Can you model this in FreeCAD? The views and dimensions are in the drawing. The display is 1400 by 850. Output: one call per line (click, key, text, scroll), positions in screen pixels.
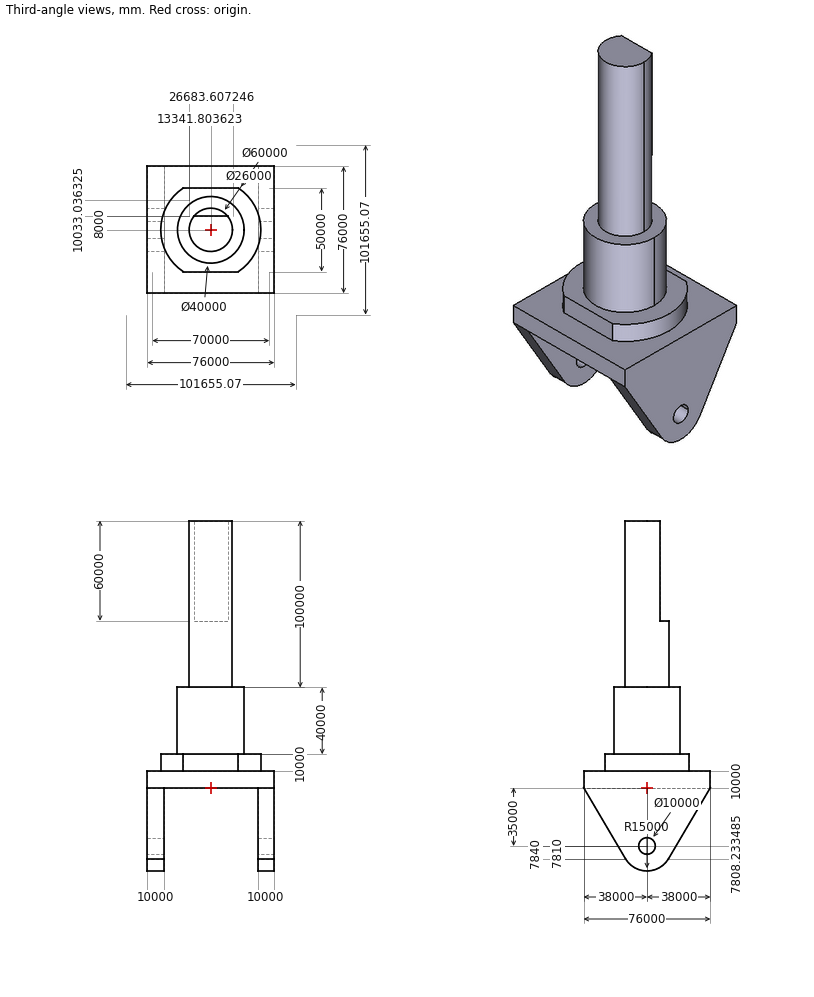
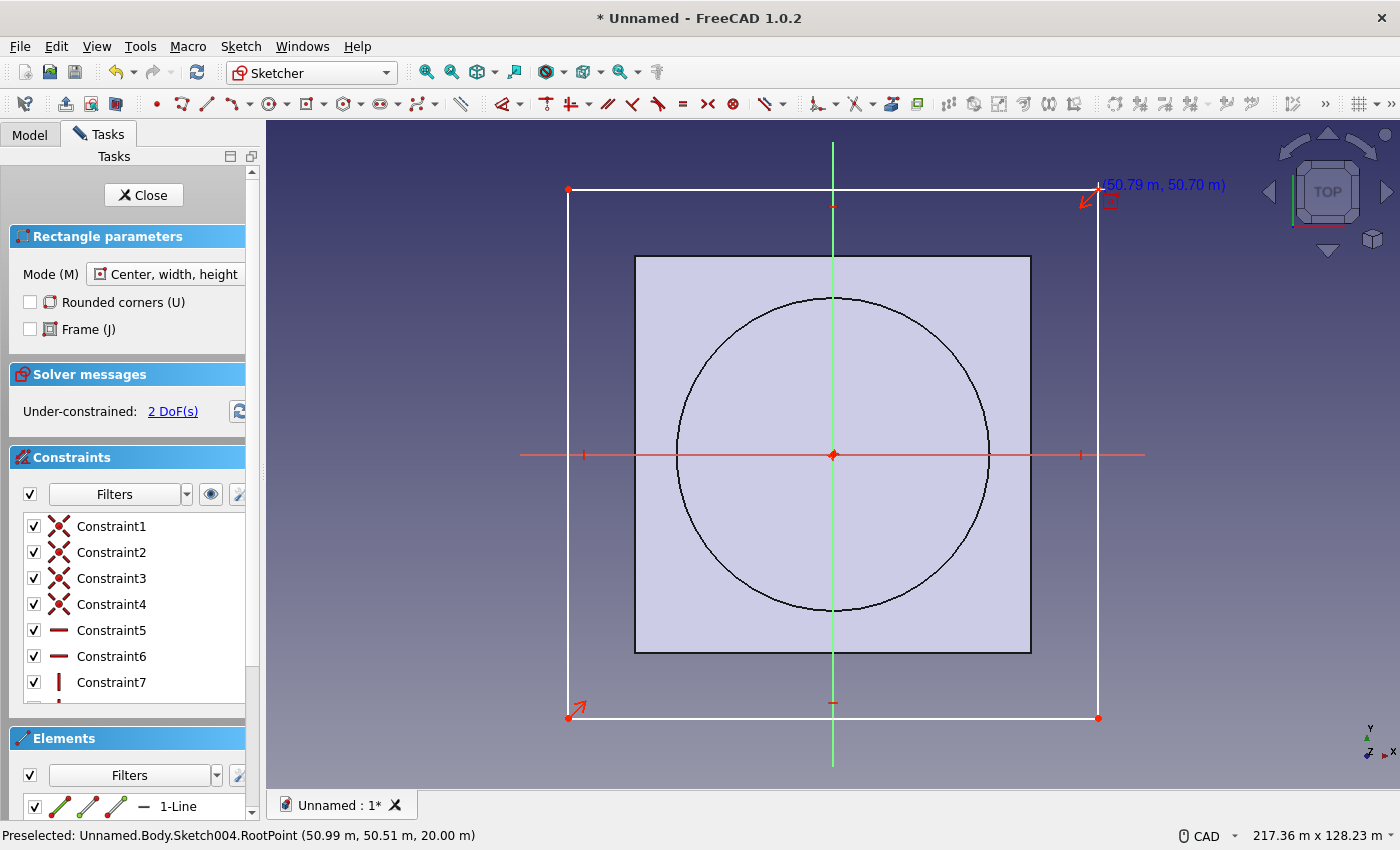
click(833, 454)
click(1016, 324)
key(Escape)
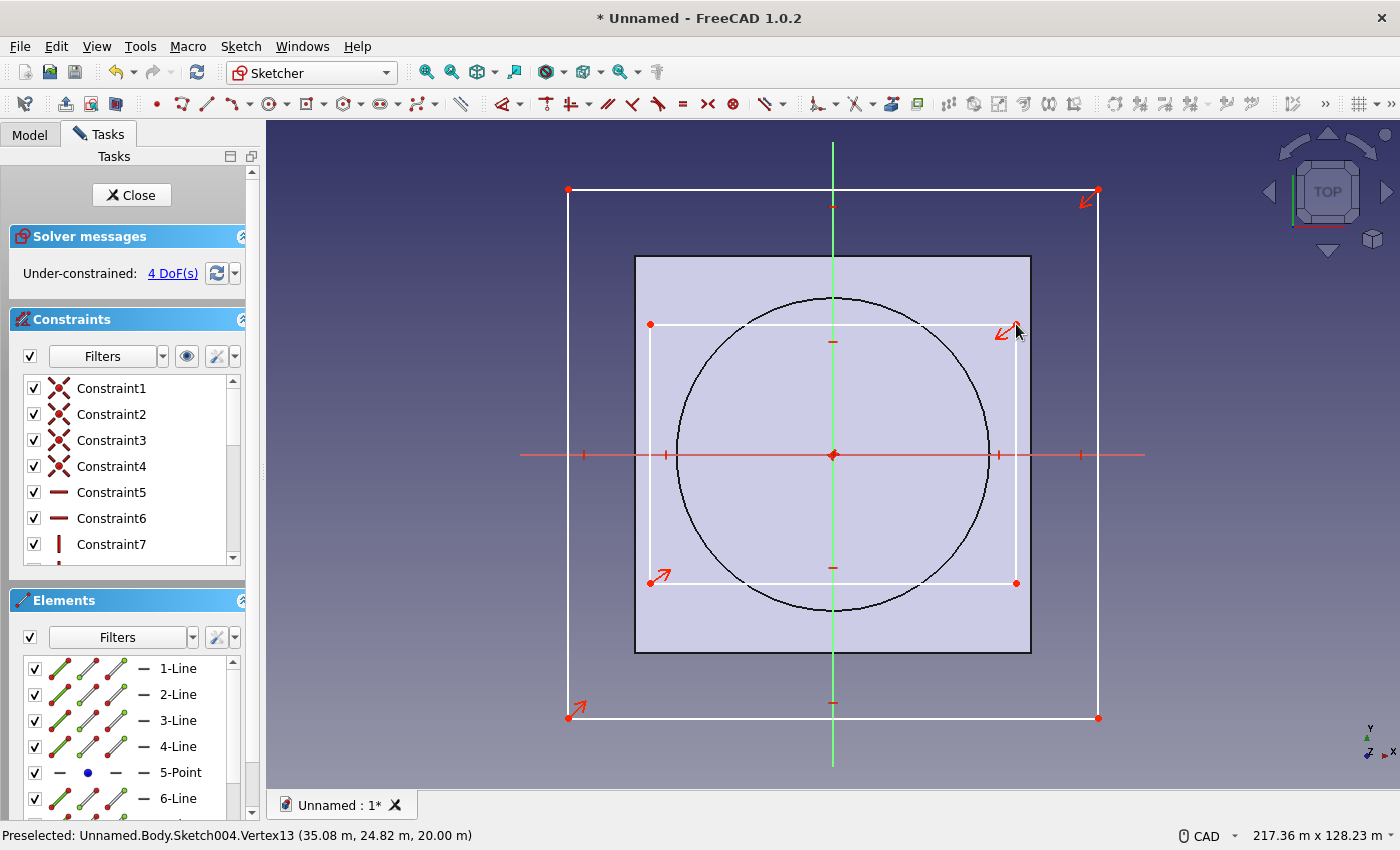
click(502, 104)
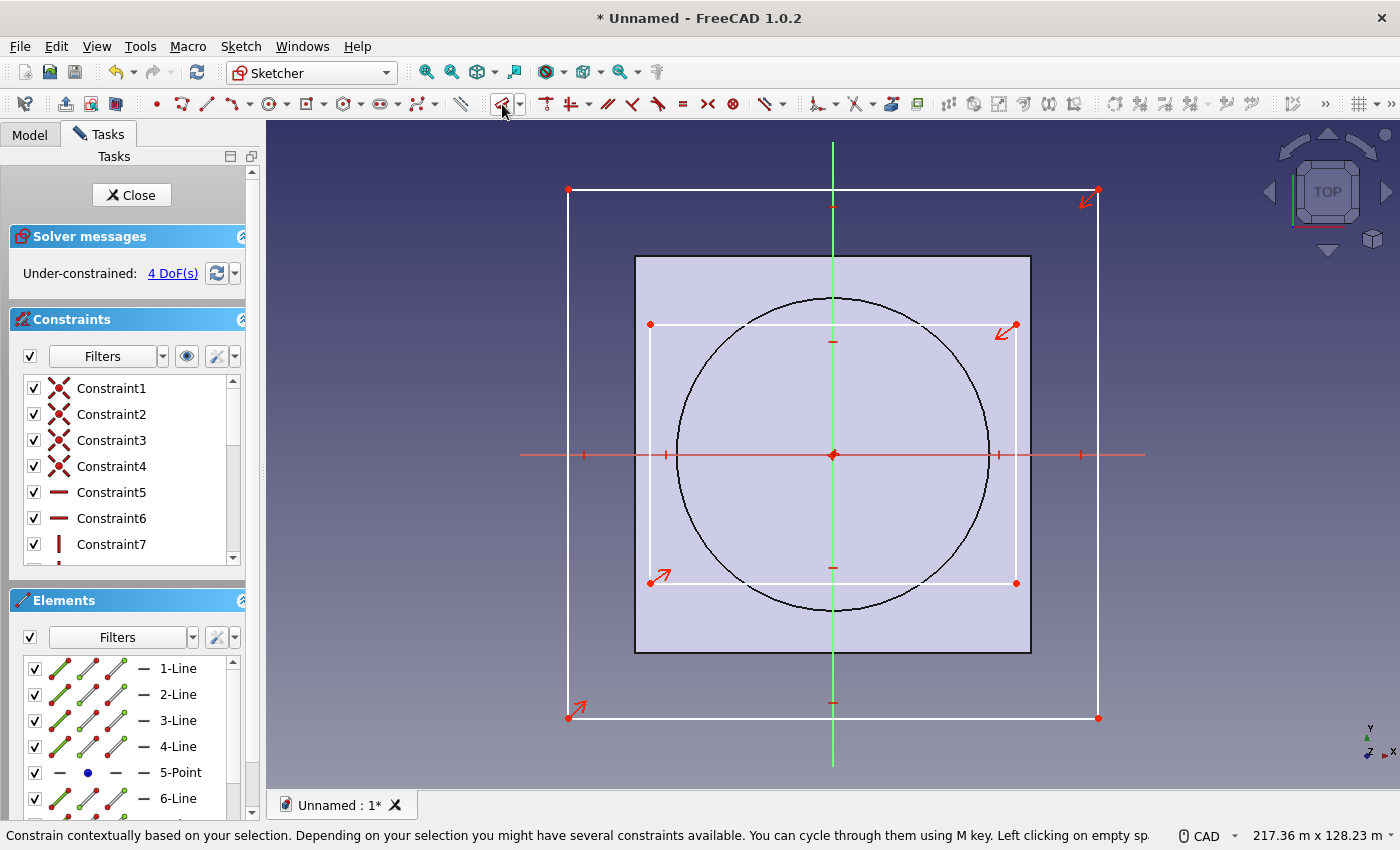
click(760, 584)
click(749, 618)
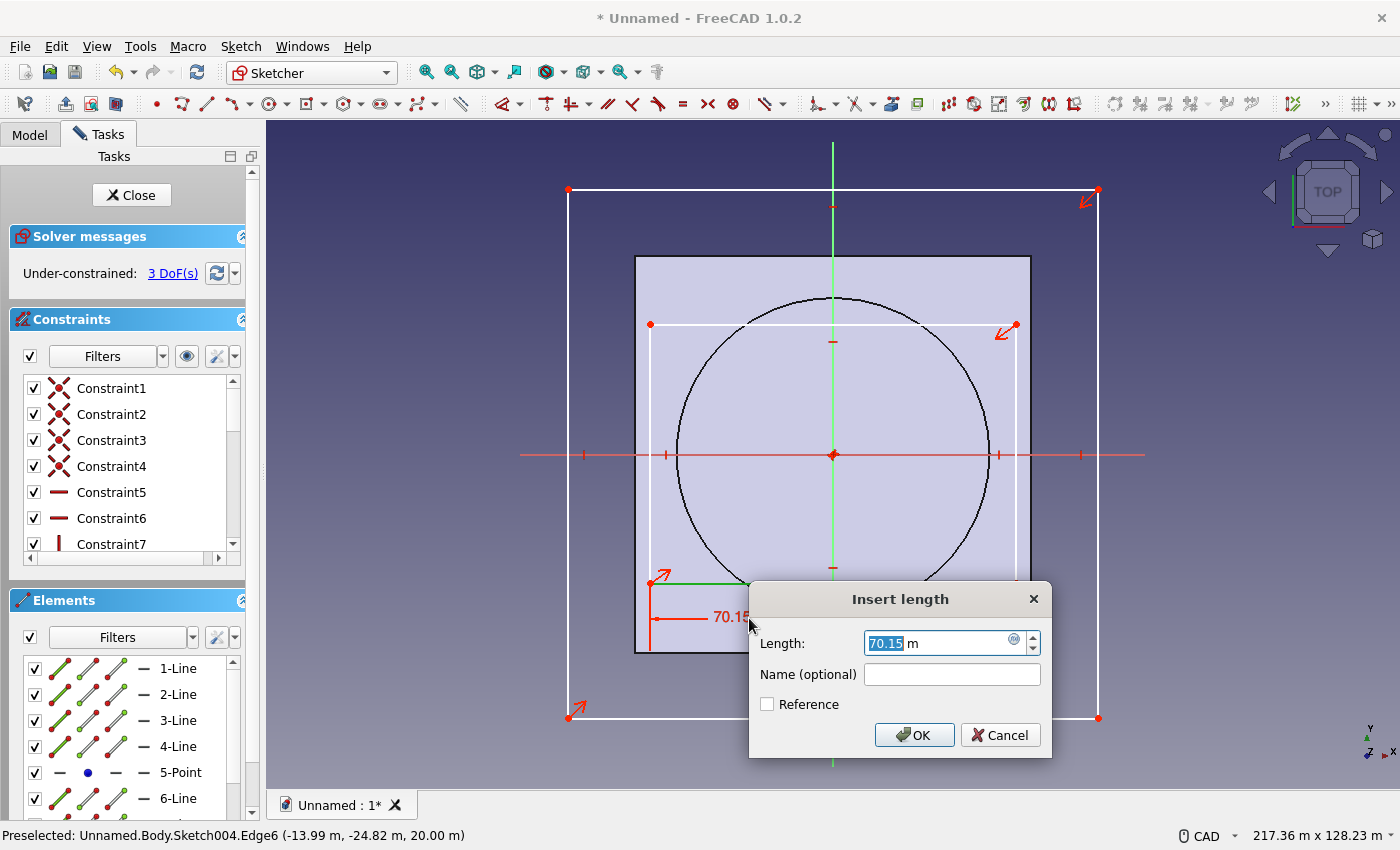
key(ctrl+a)
text(70000 mm)
key(Return)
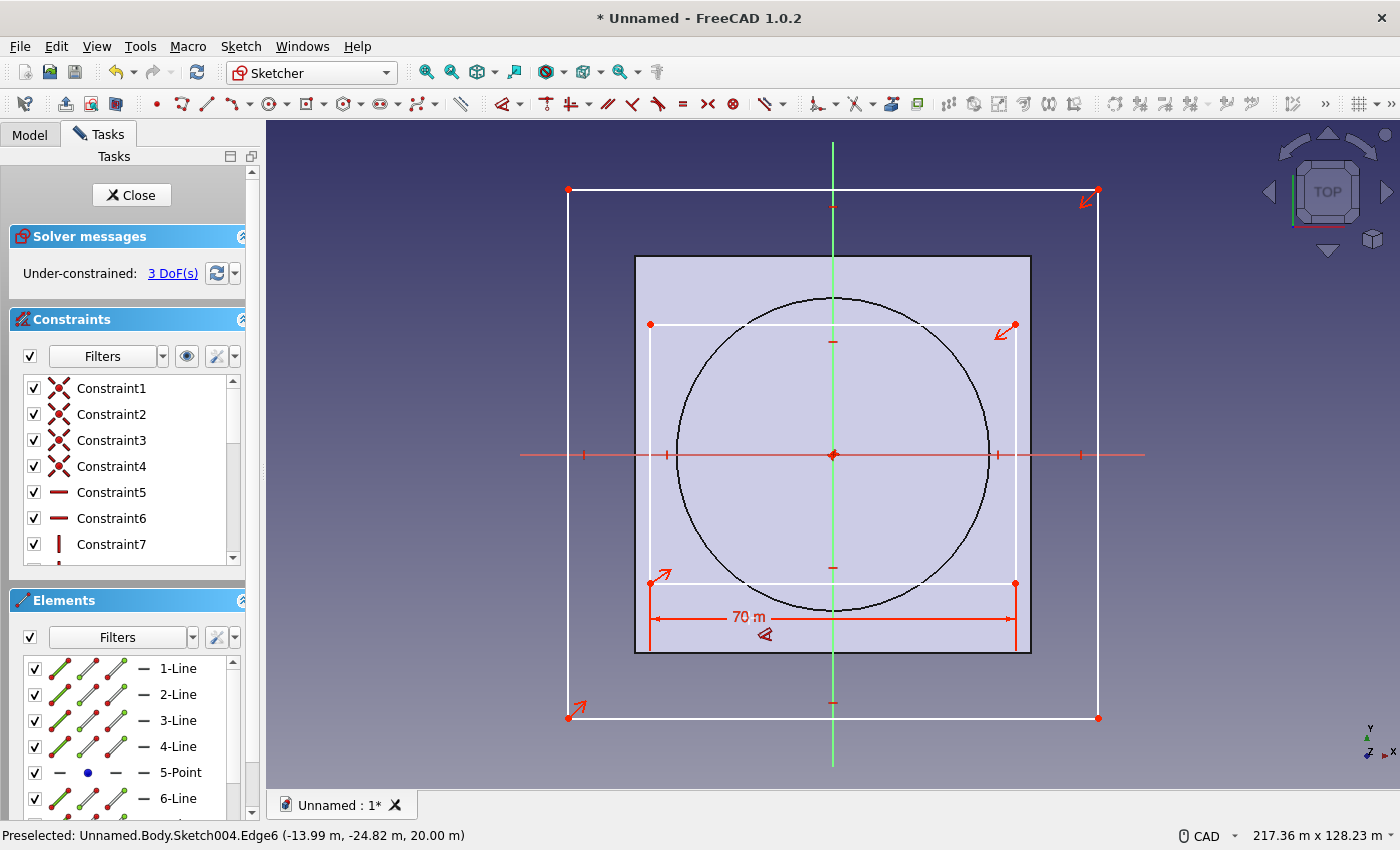
click(1016, 506)
click(1050, 395)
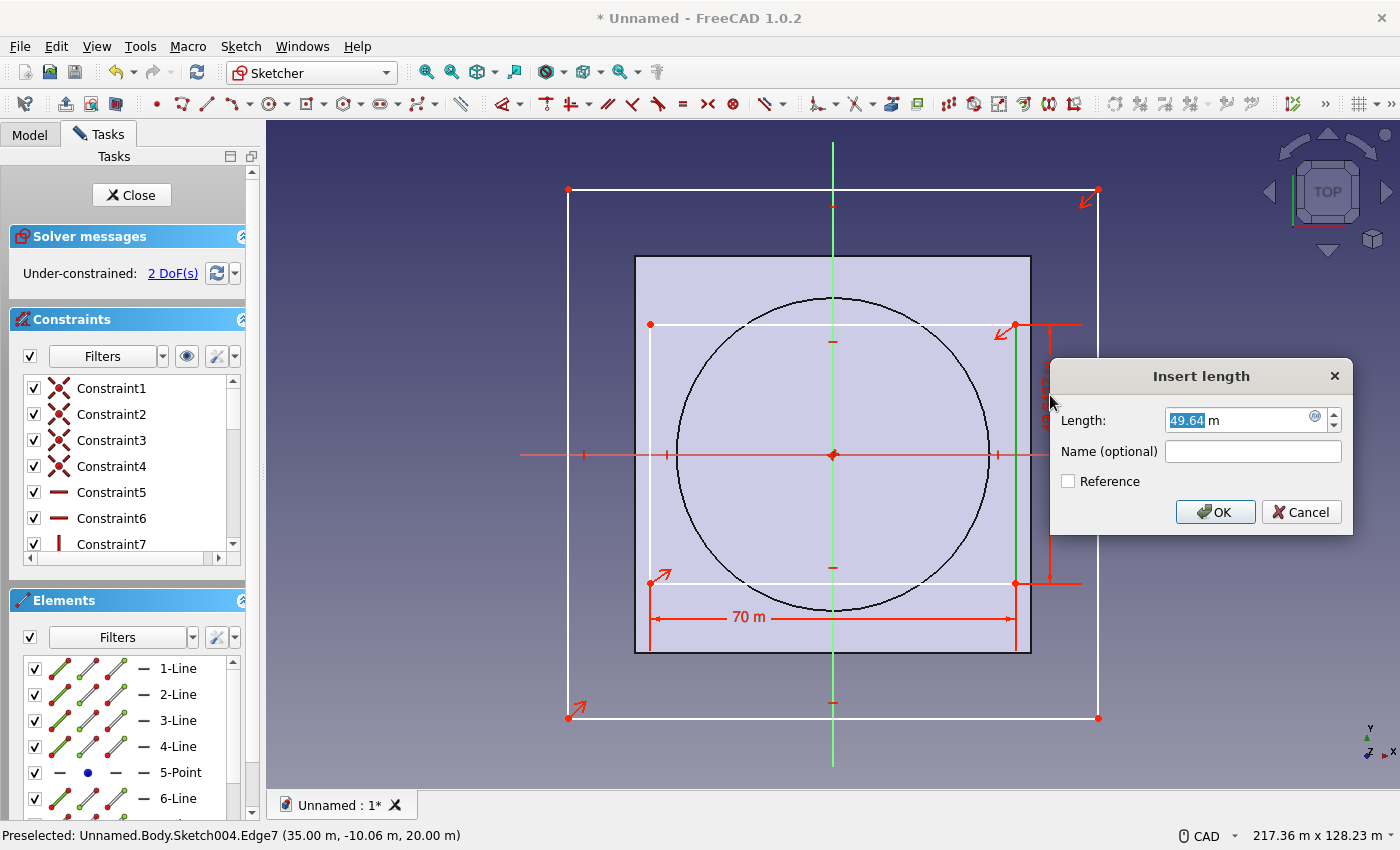
key(ctrl+a)
text(50000 mm)
key(Return)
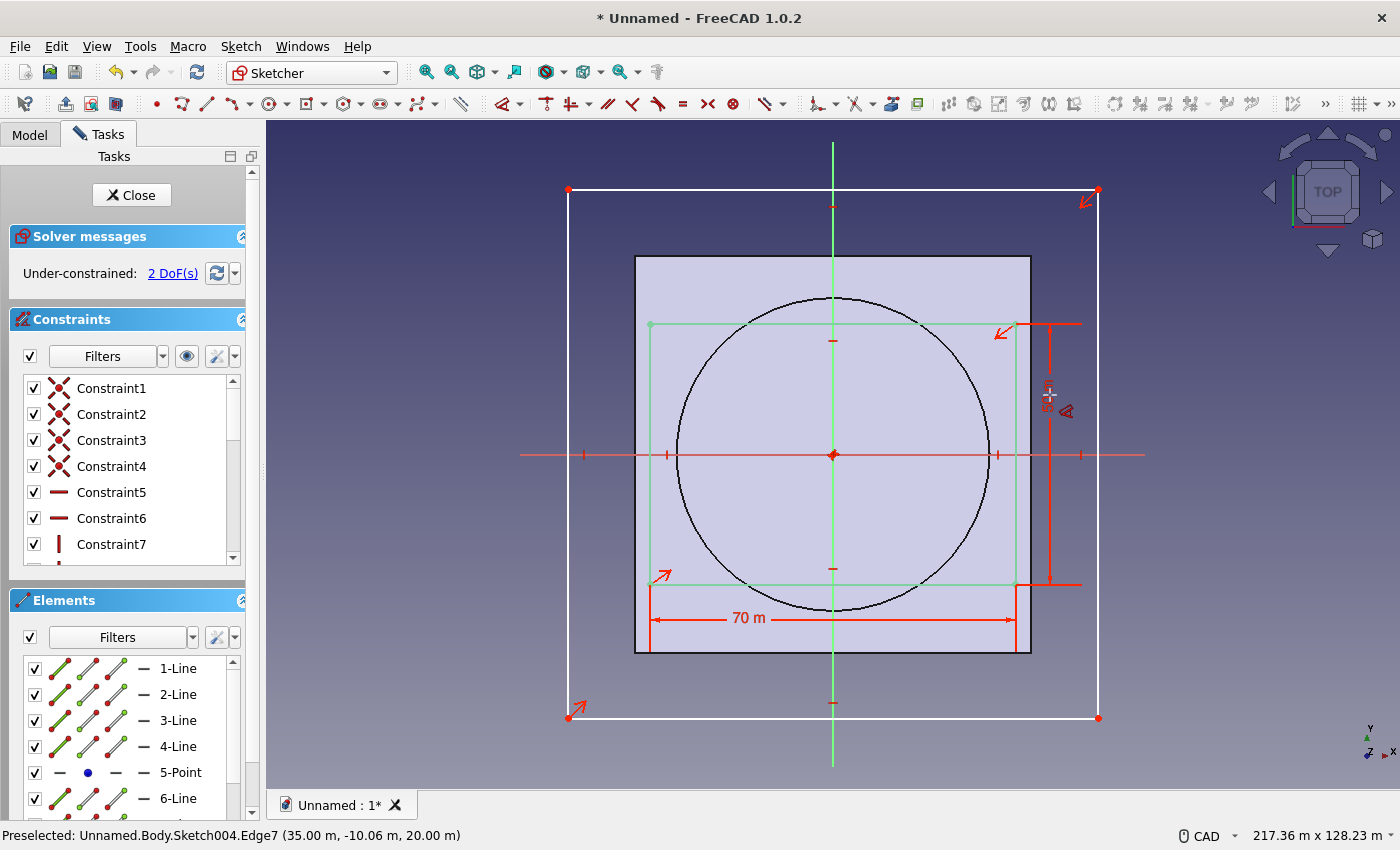
click(727, 719)
click(711, 753)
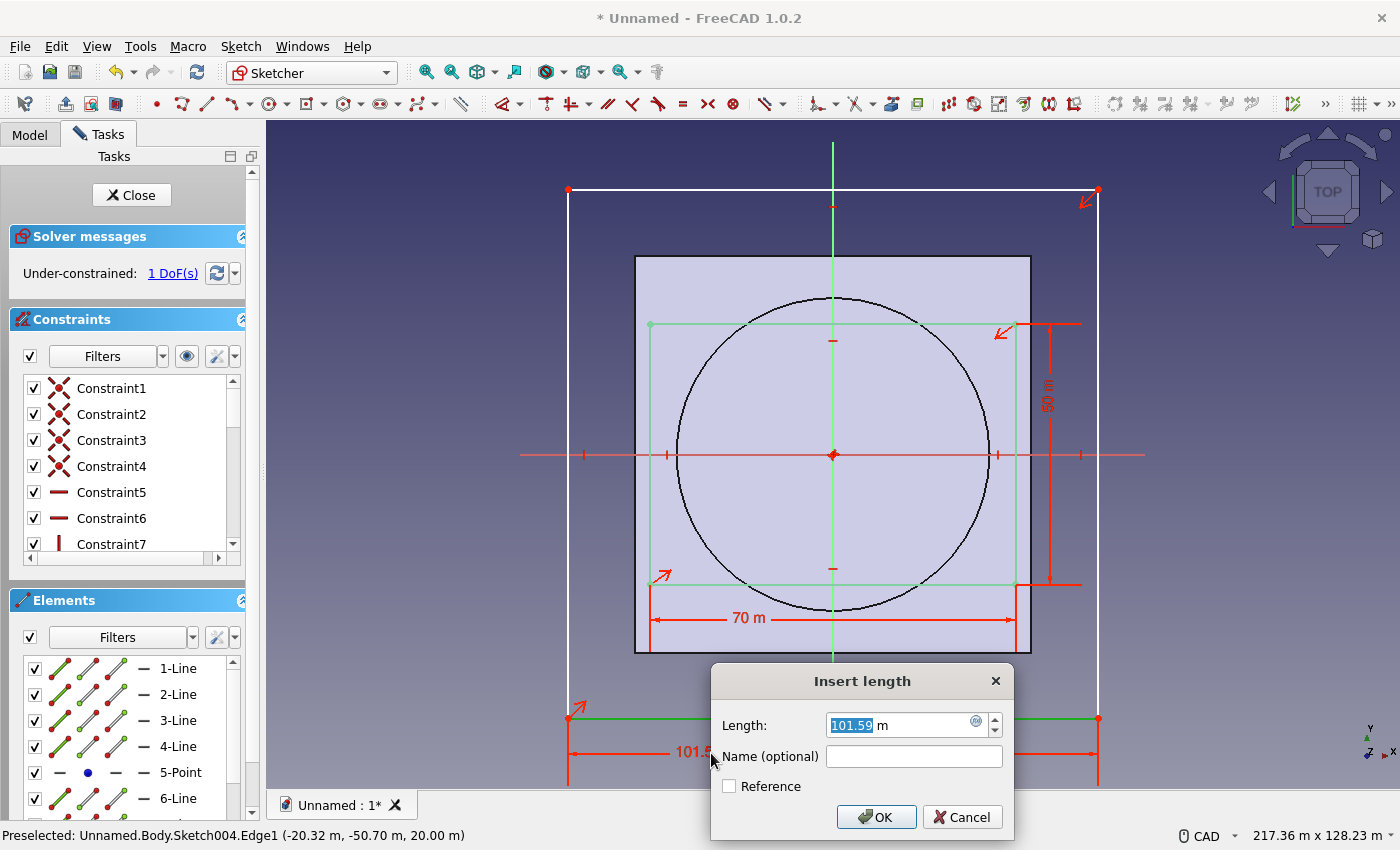
key(ctrl+a)
text(101655.07 mm)
key(Return)